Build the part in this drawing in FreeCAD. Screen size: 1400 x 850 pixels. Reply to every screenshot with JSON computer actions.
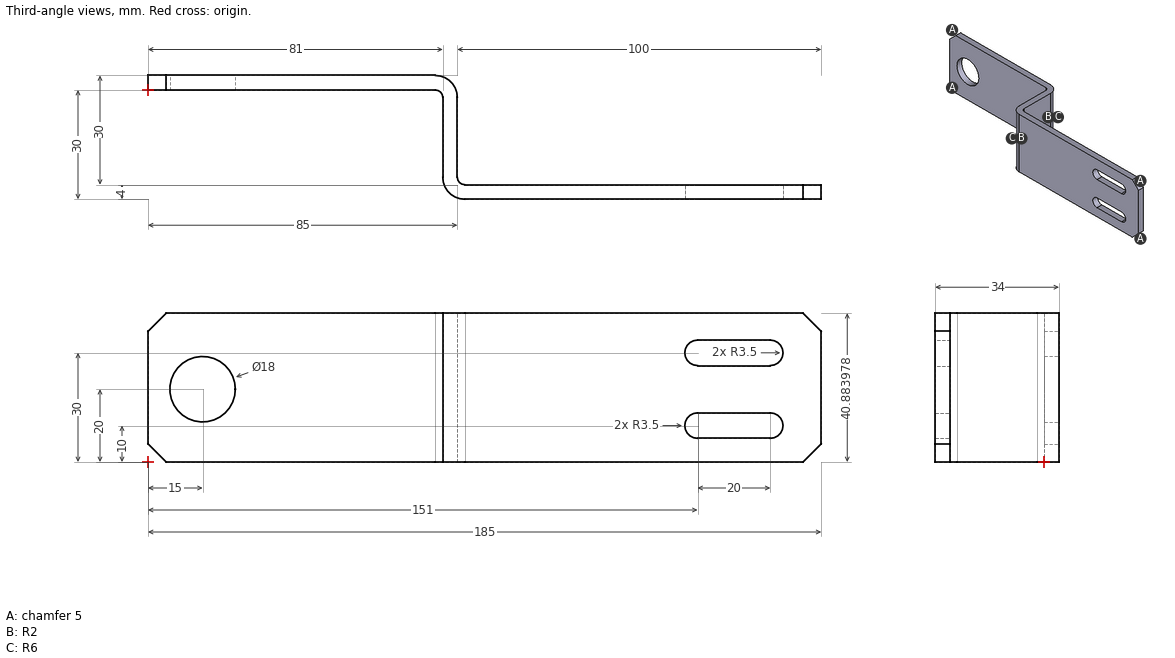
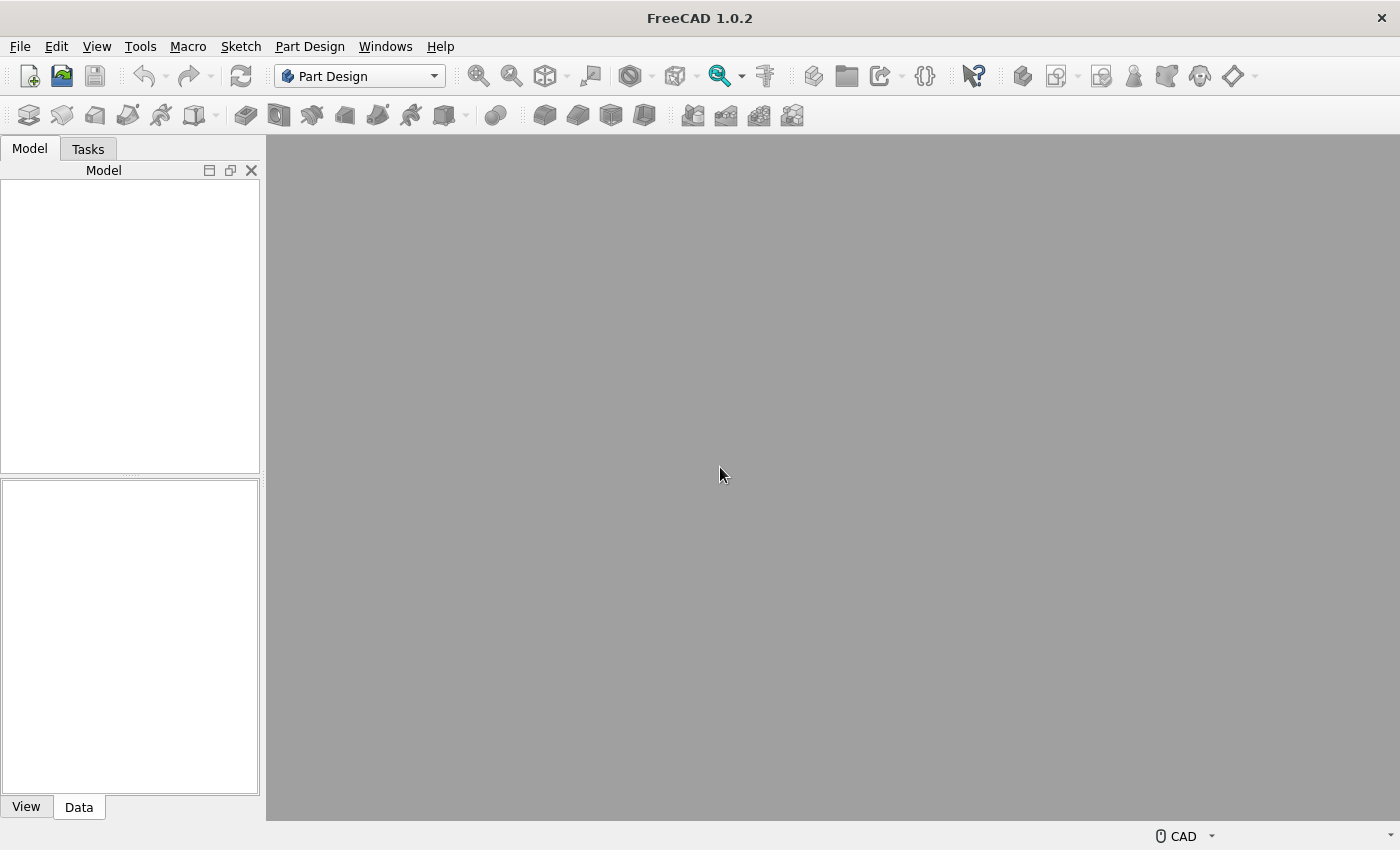
{"action": "left_click", "coordinate": [29, 76]}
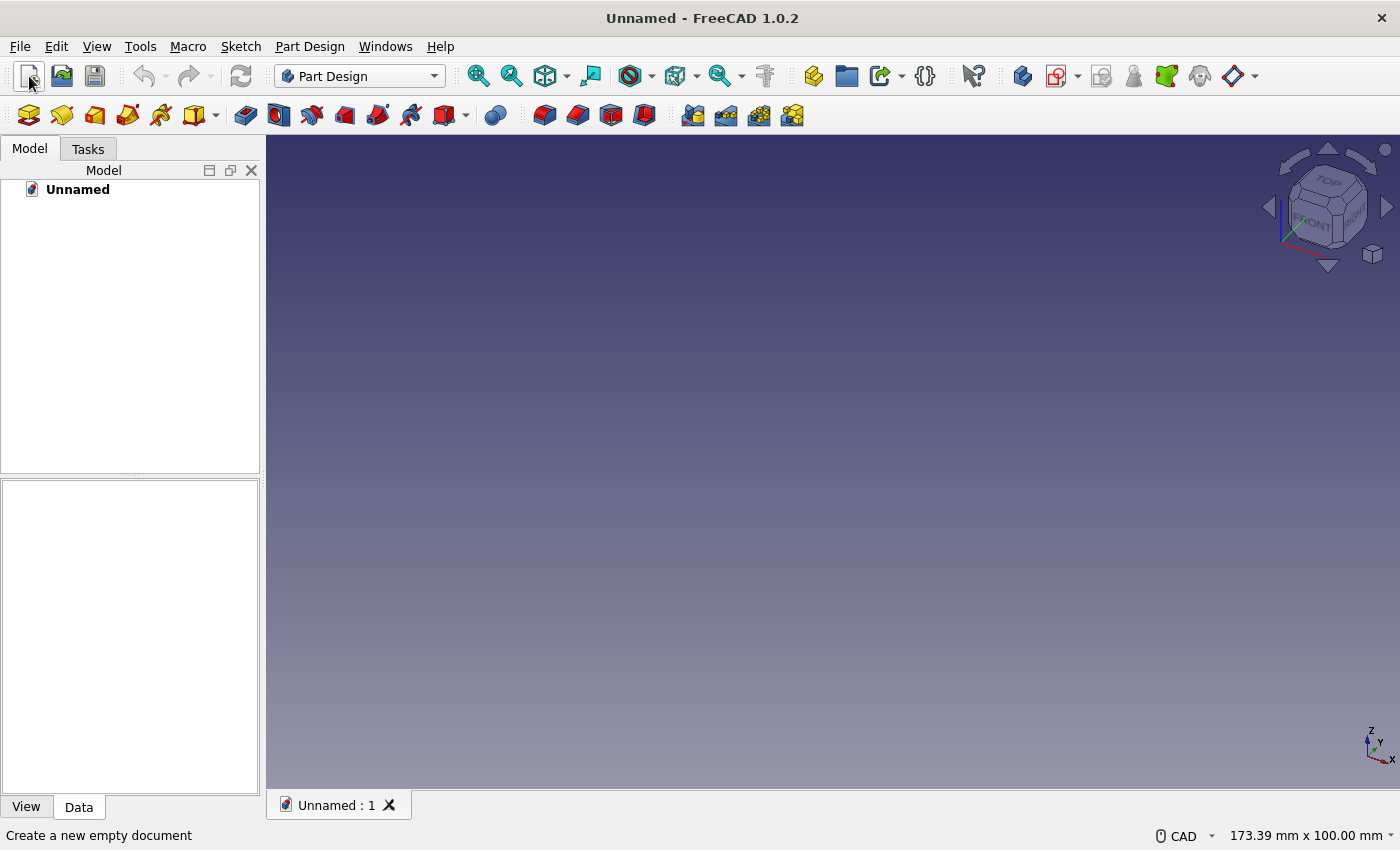
{"action": "left_click", "coordinate": [1023, 76]}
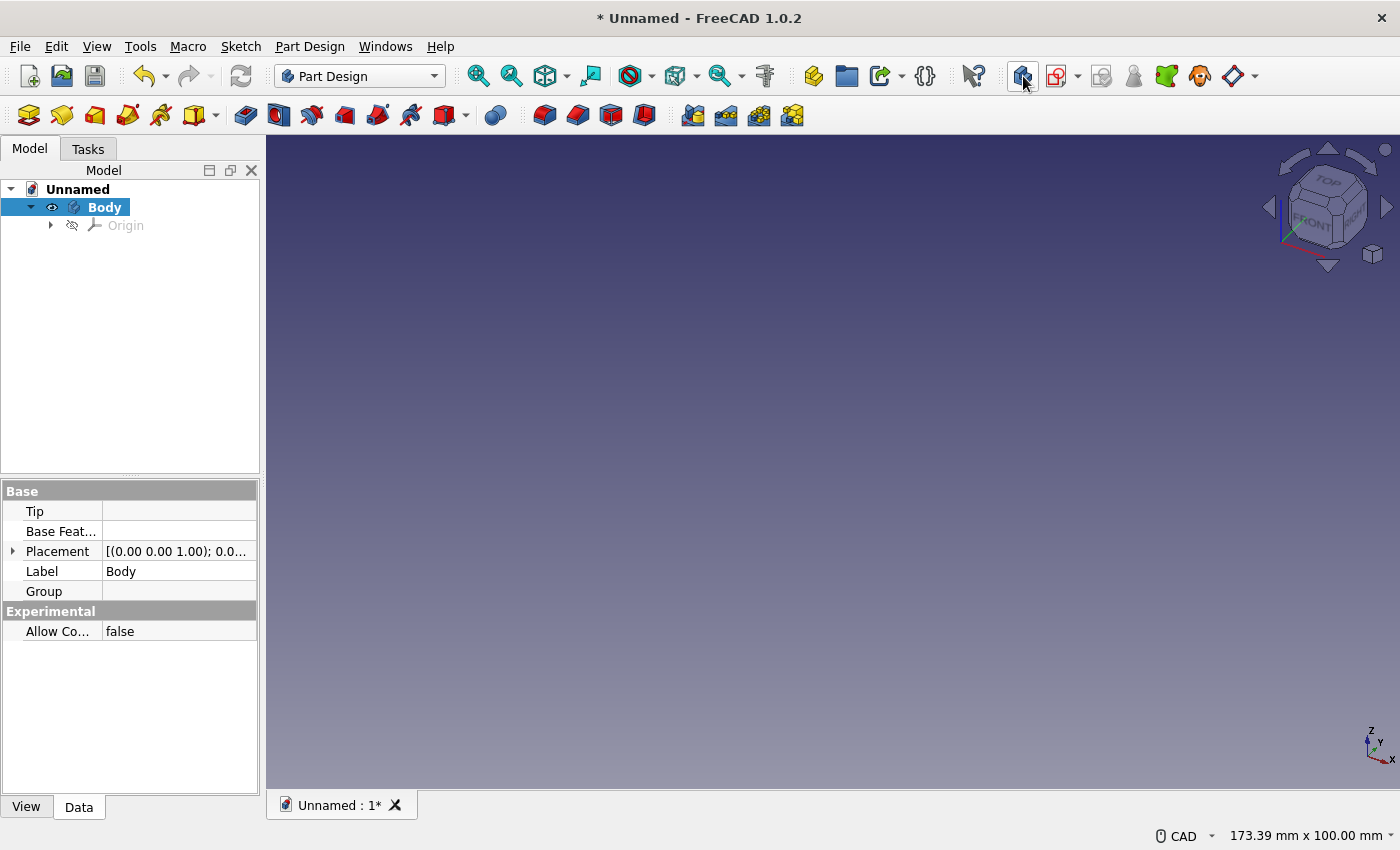
{"action": "left_click", "coordinate": [51, 225]}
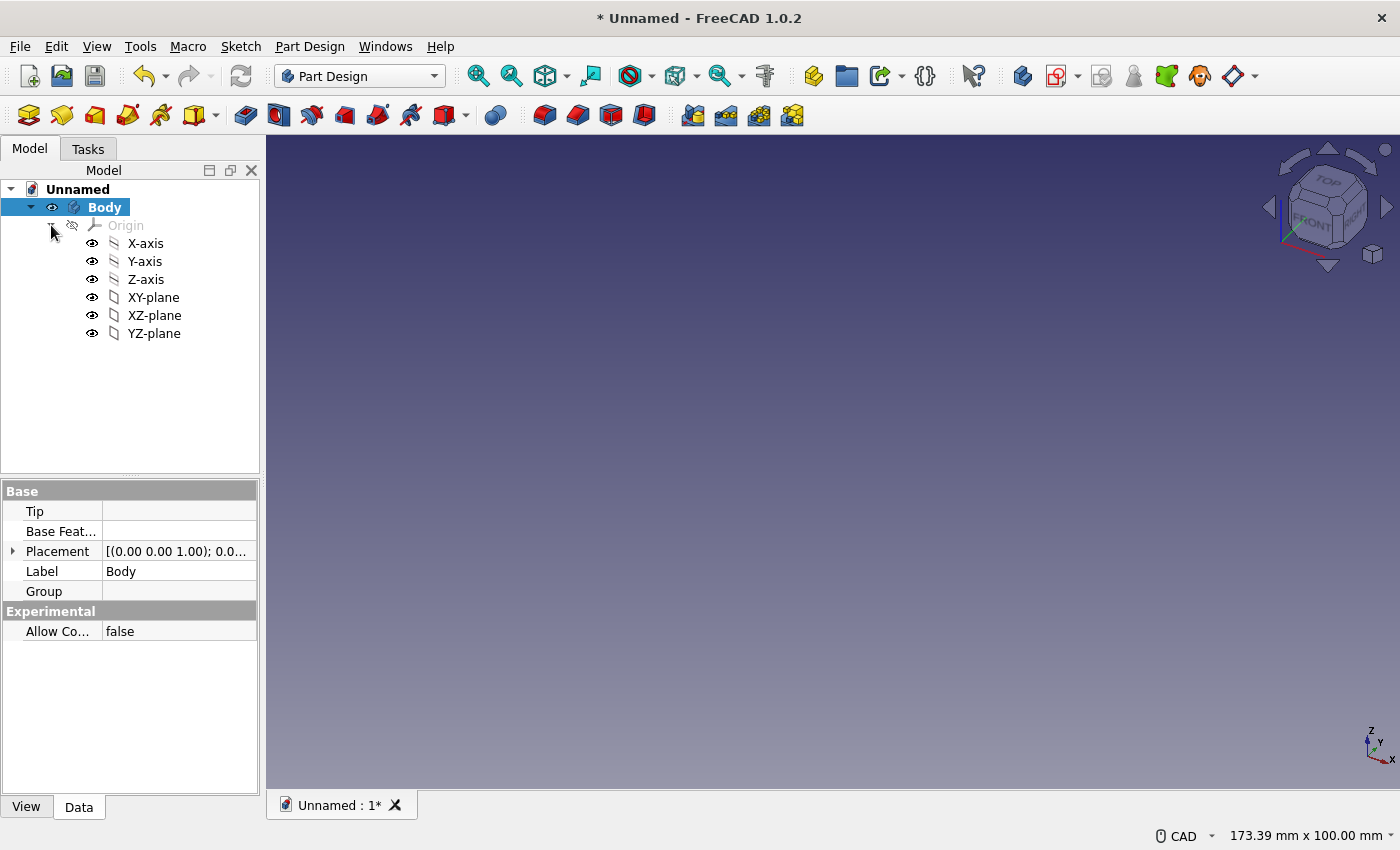
{"action": "left_click", "coordinate": [137, 315]}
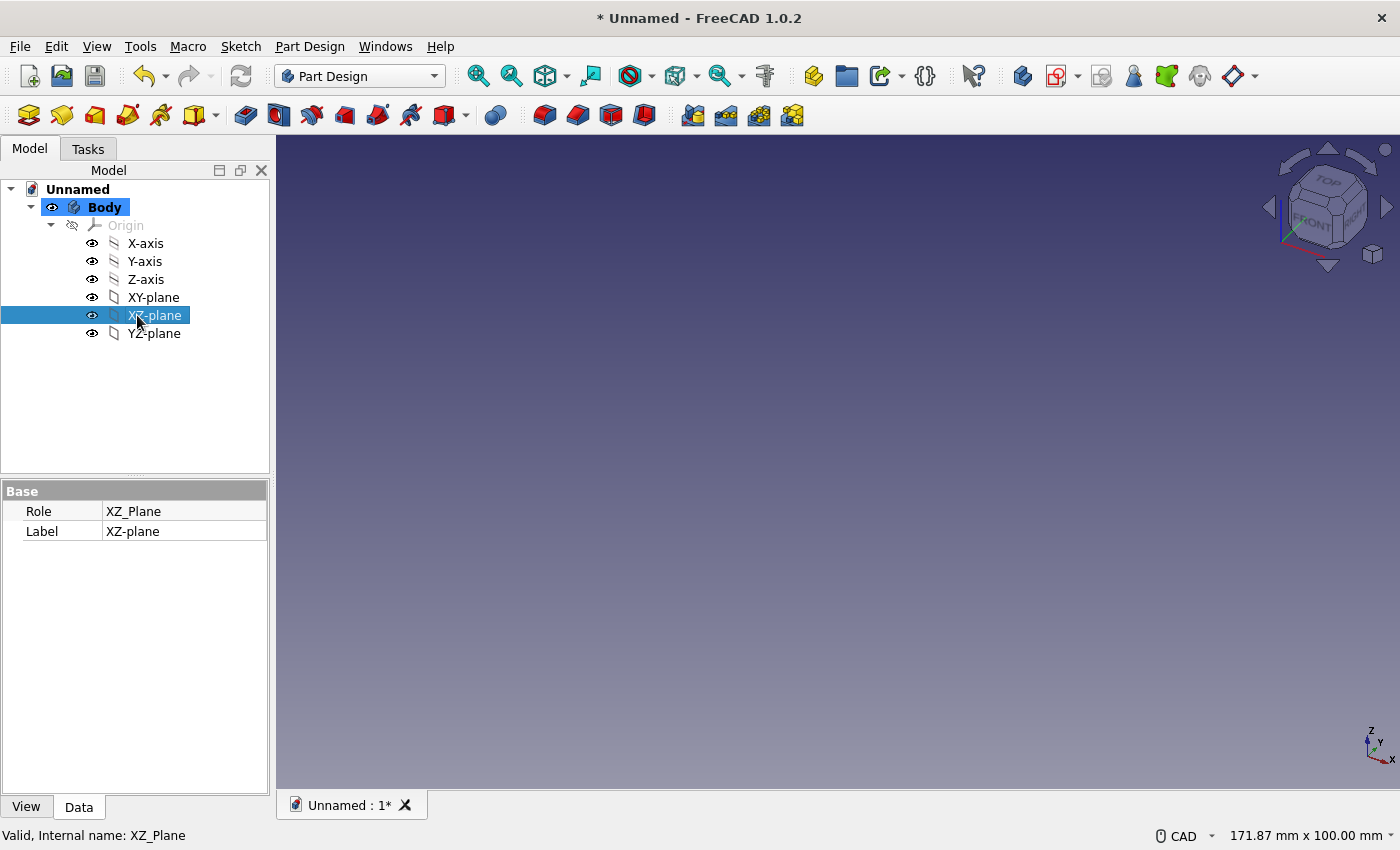
{"action": "left_click", "coordinate": [1232, 76]}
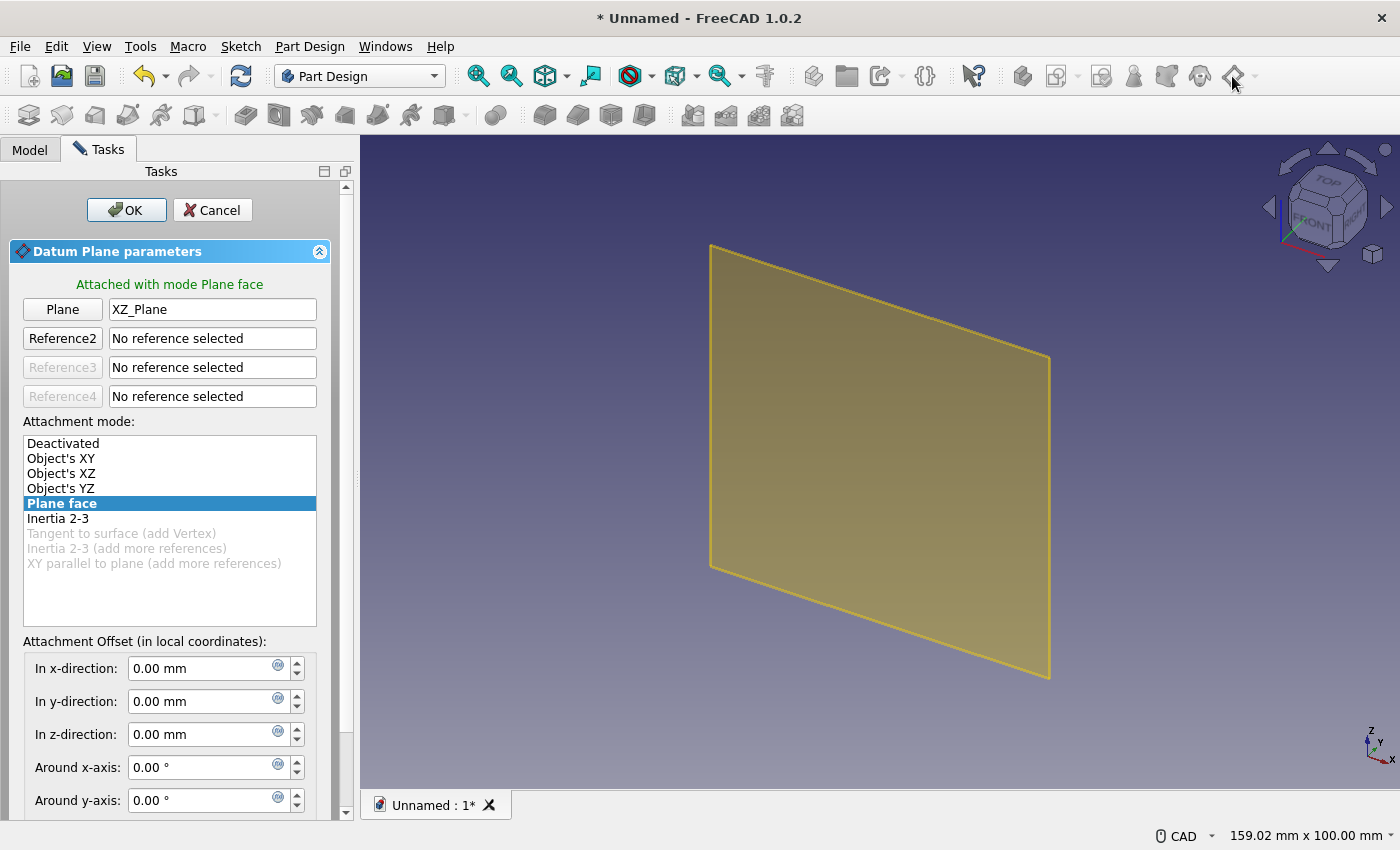
{"action": "triple_click", "coordinate": [210, 734]}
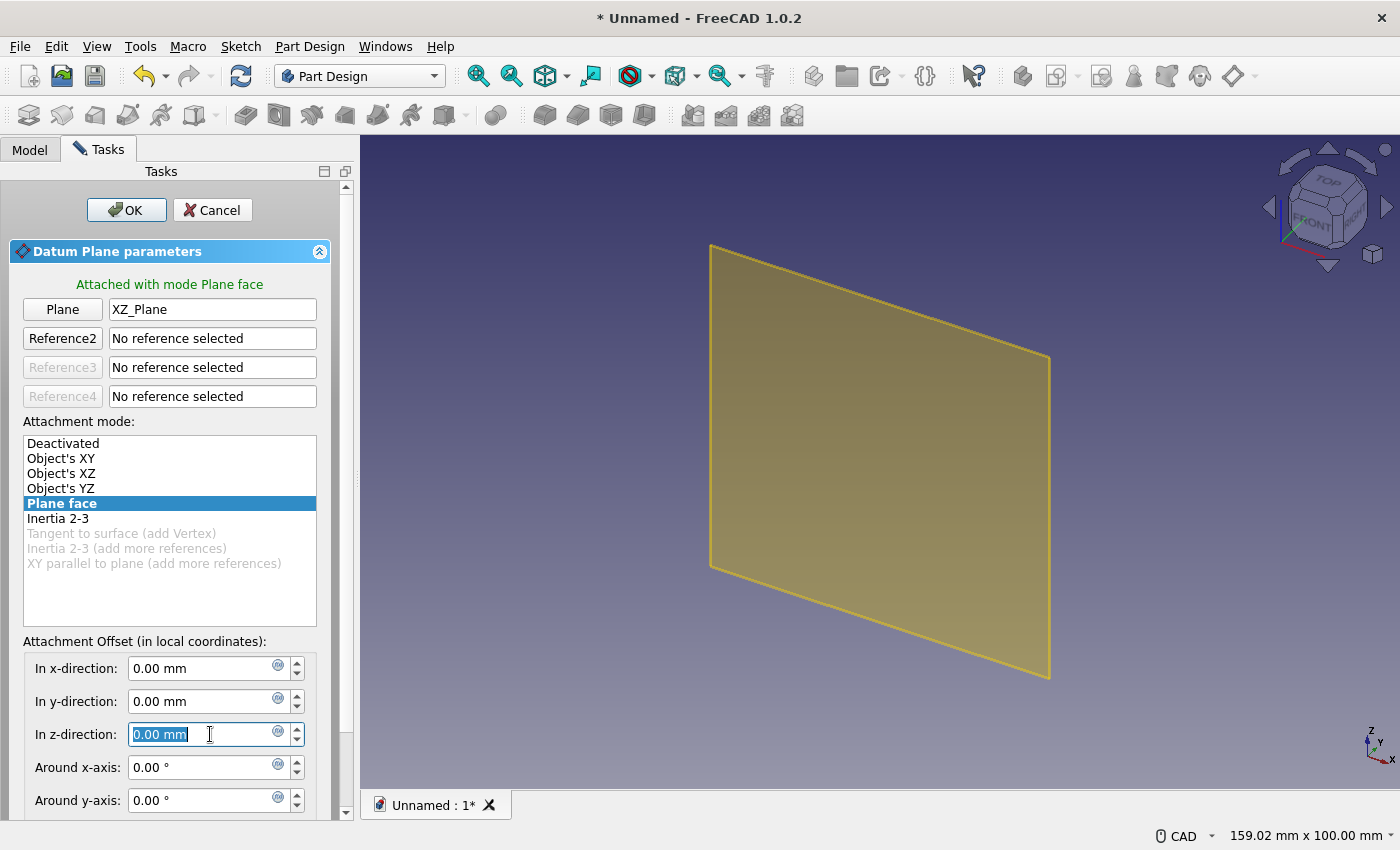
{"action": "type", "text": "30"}
{"action": "key", "text": "Tab"}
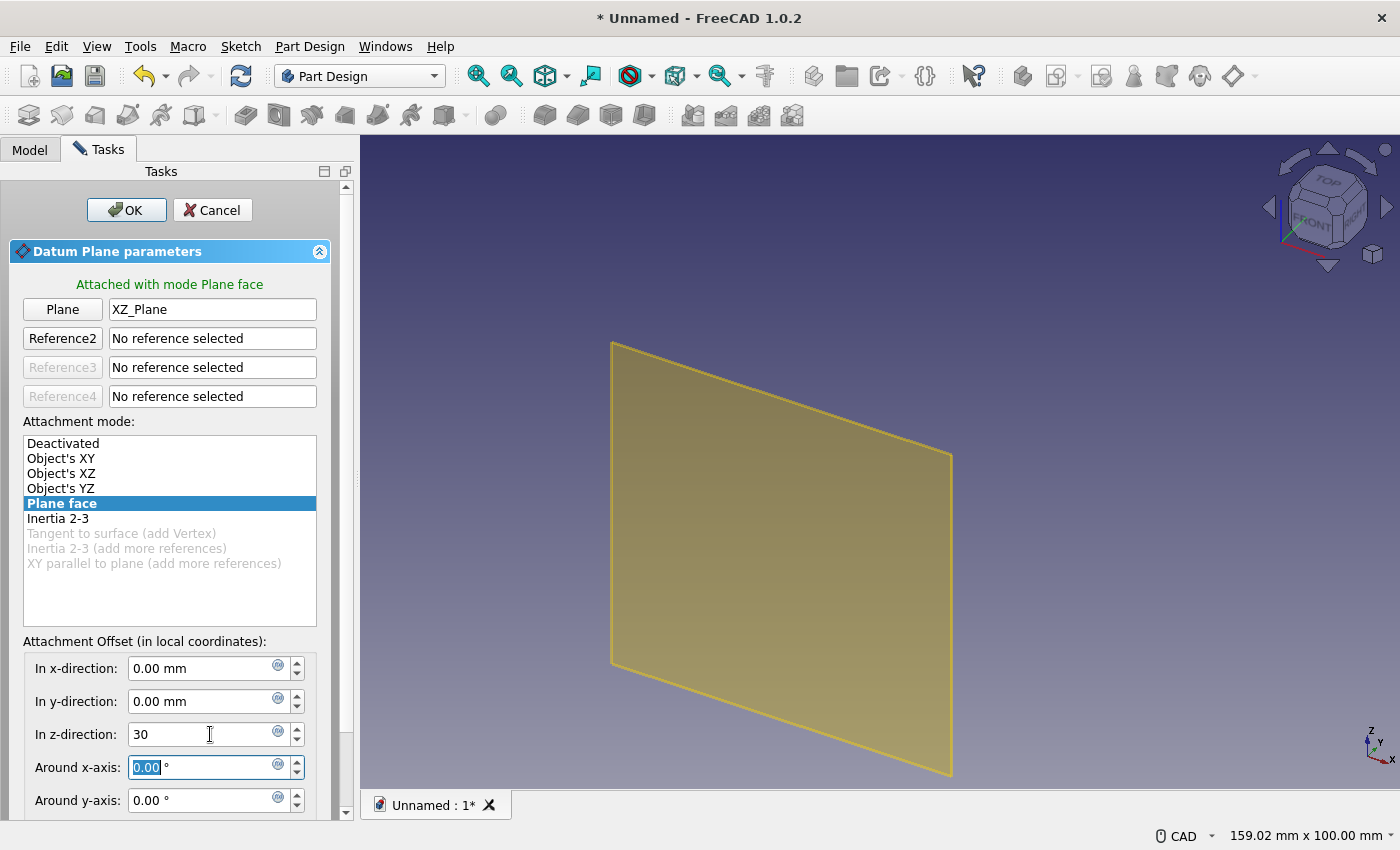
{"action": "left_click", "coordinate": [127, 210]}